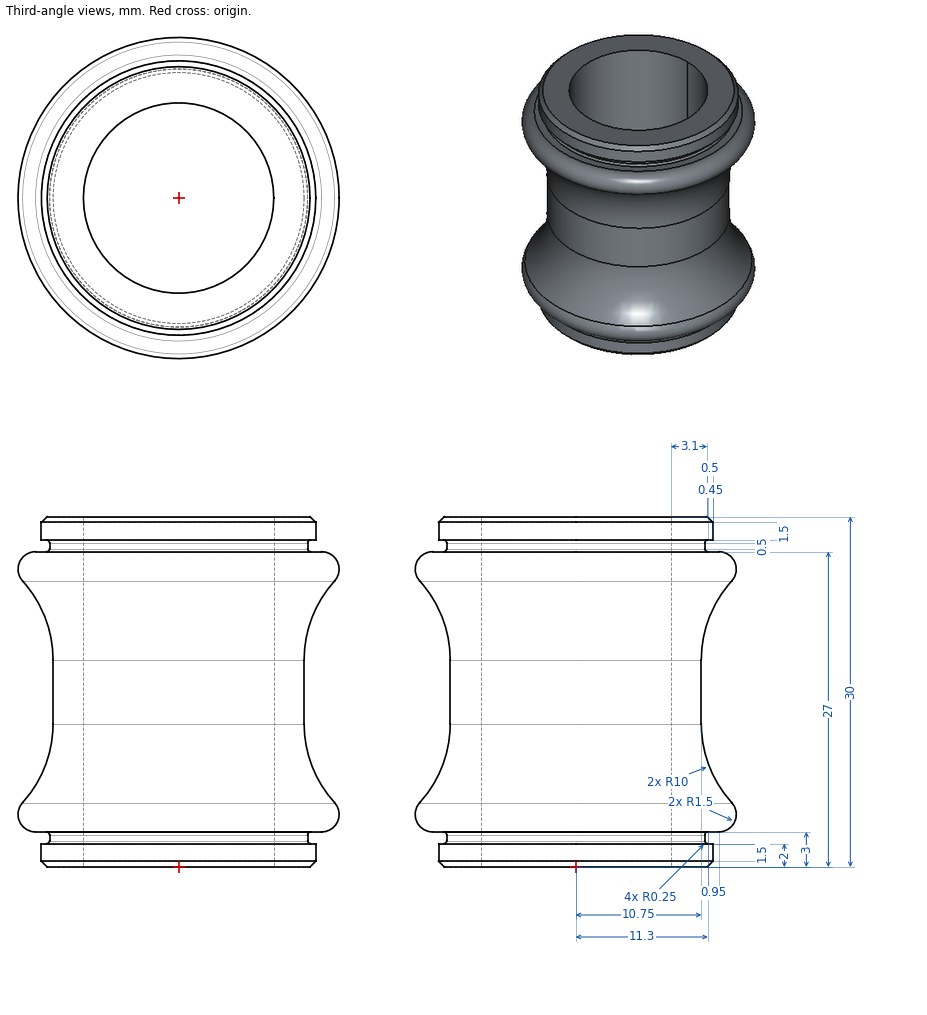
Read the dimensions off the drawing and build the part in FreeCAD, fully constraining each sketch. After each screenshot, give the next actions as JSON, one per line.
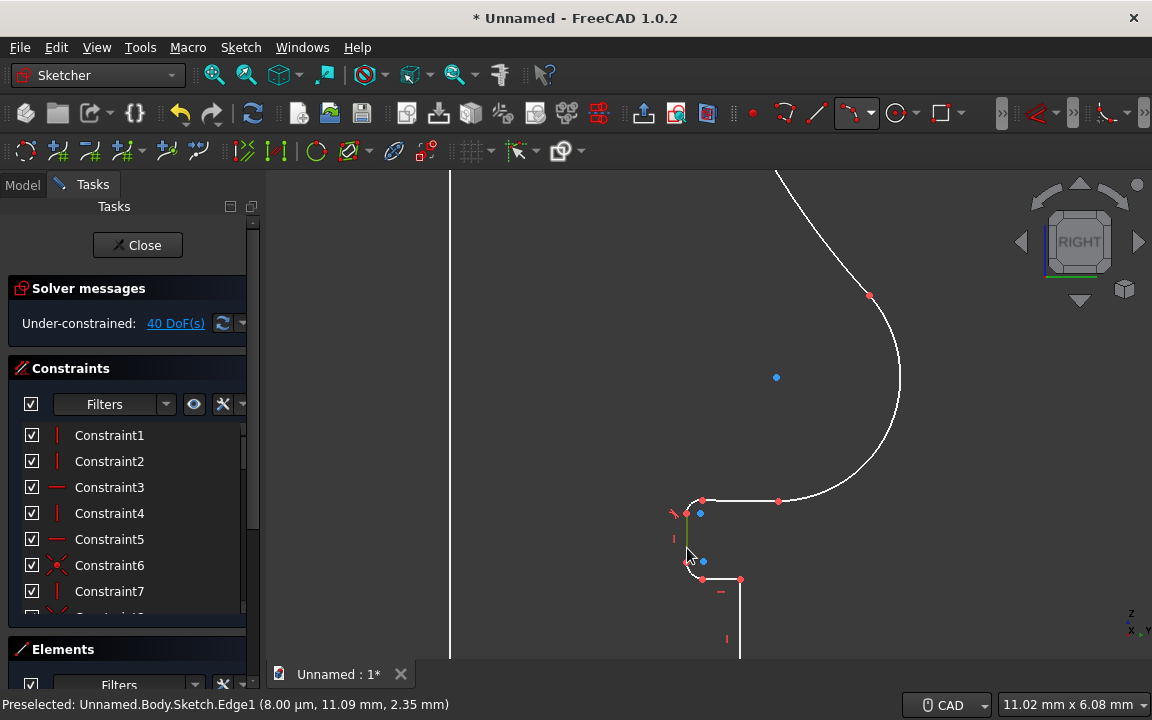
{"action": "left_click", "coordinate": [692, 574]}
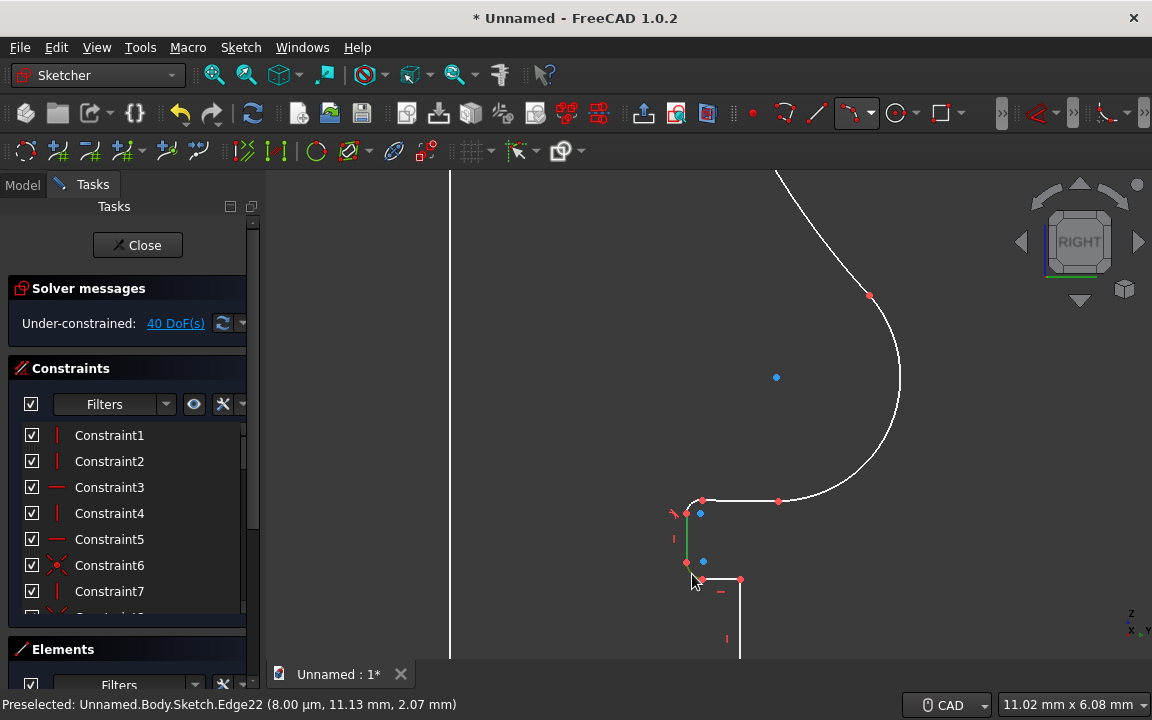
{"action": "key", "text": "t"}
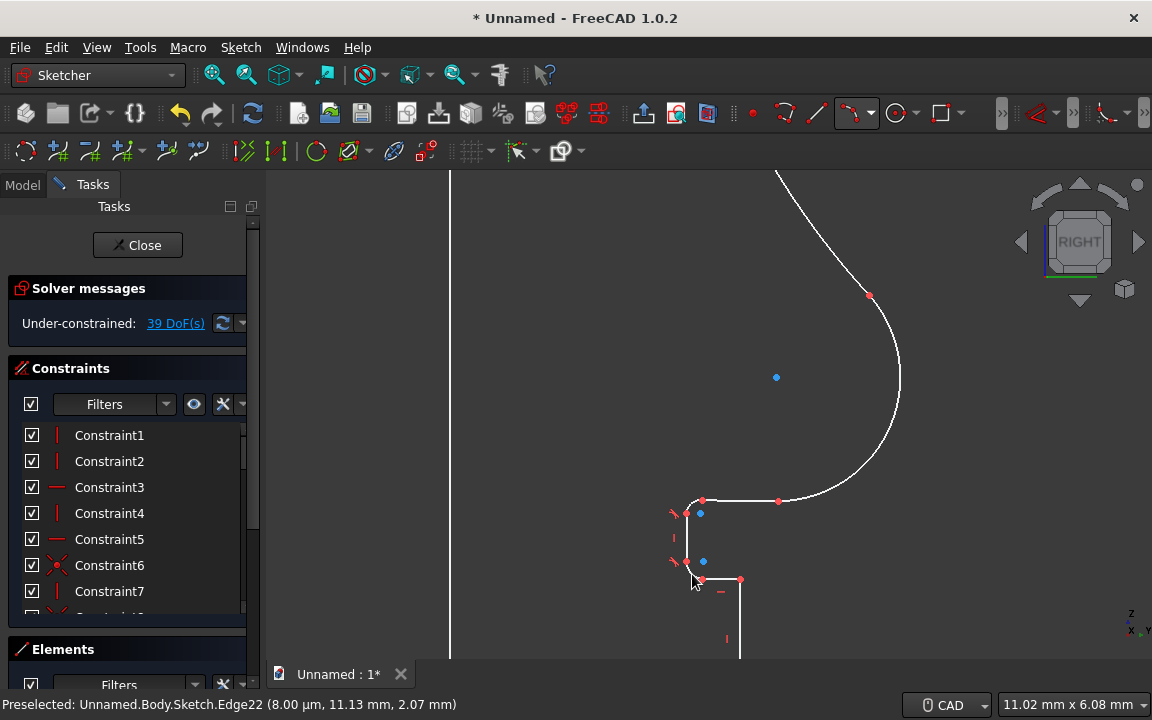
{"action": "left_click", "coordinate": [725, 501]}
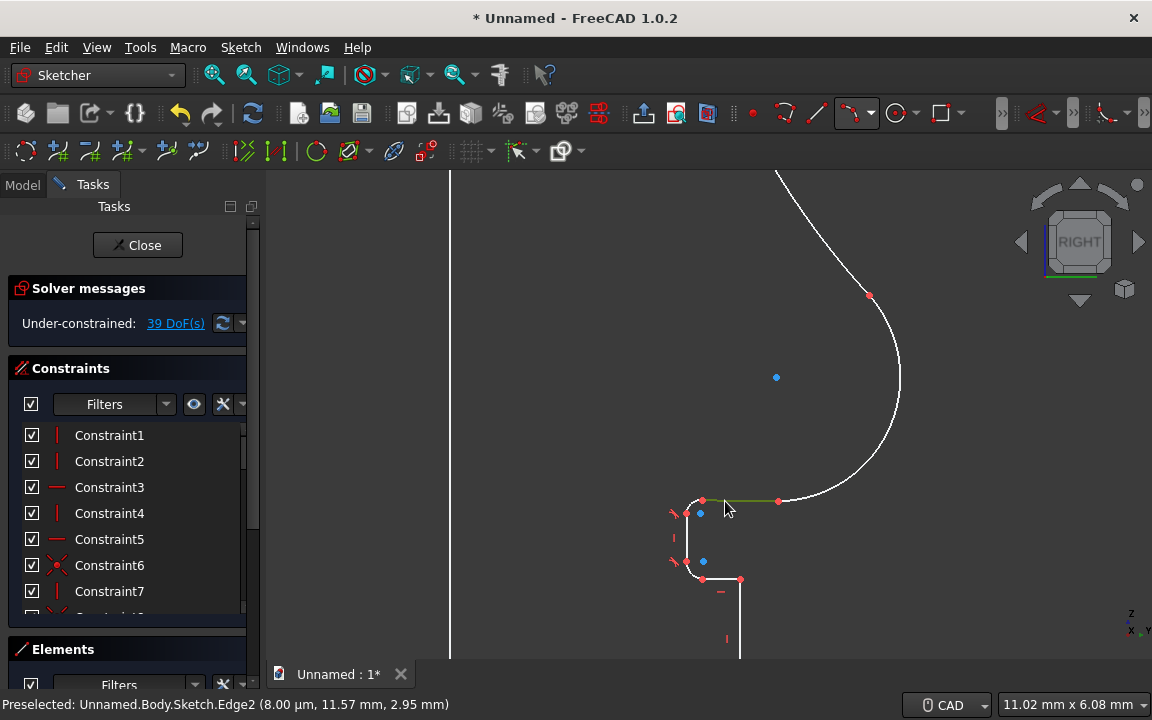
{"action": "left_click", "coordinate": [692, 503]}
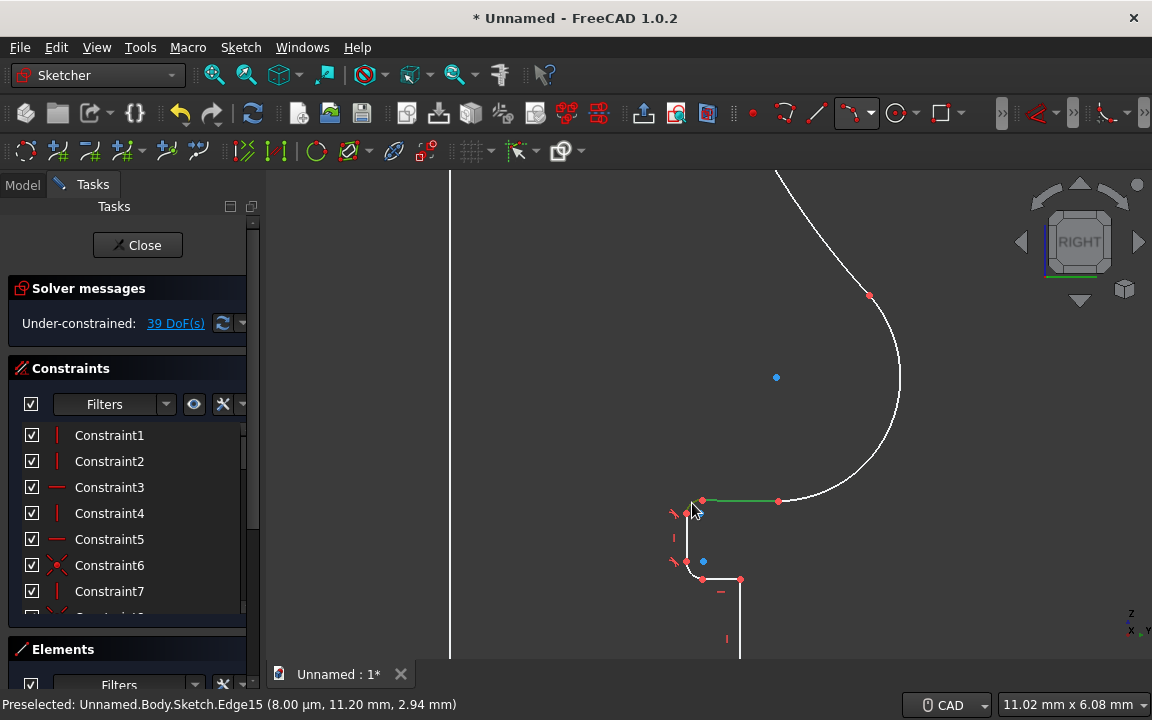
{"action": "key", "text": "t"}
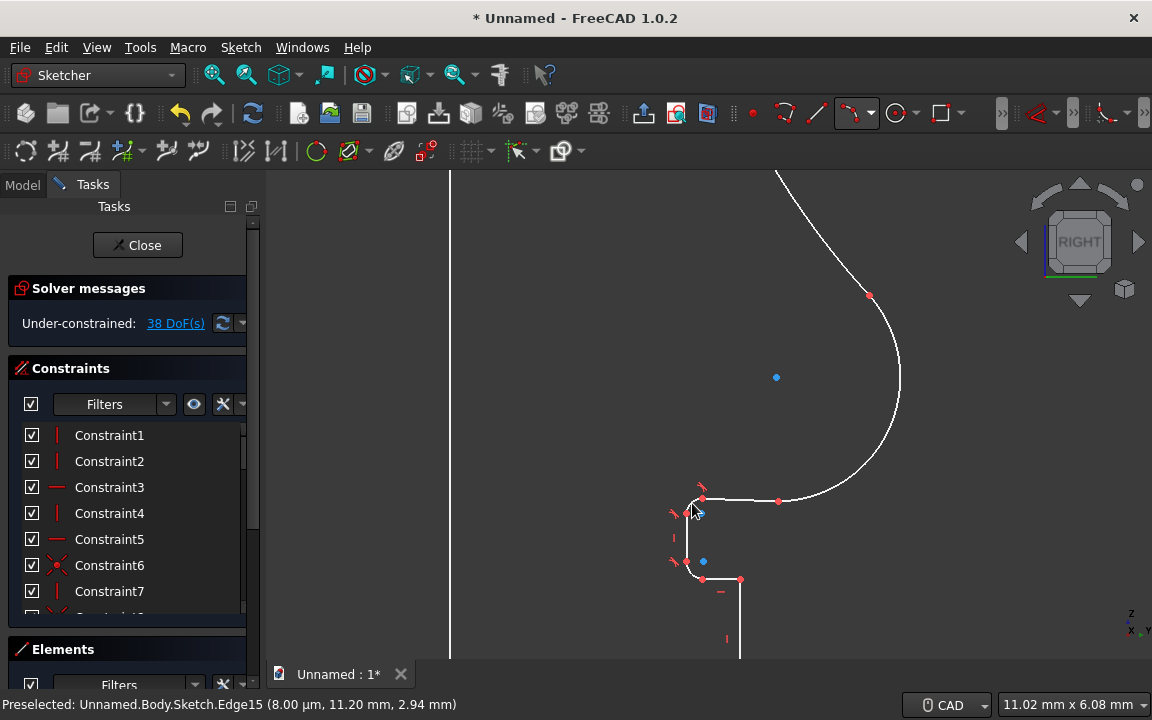
{"action": "left_click", "coordinate": [725, 499]}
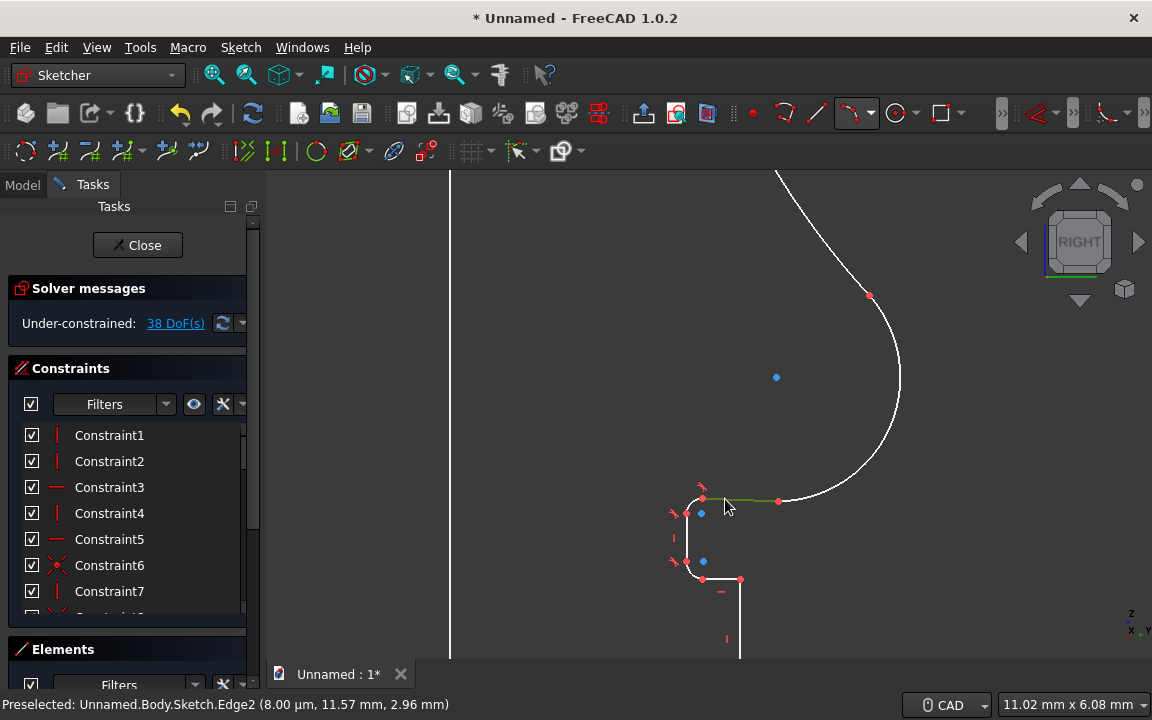
{"action": "scroll", "coordinate": [687, 553], "scroll_direction": "down", "scroll_amount": 10}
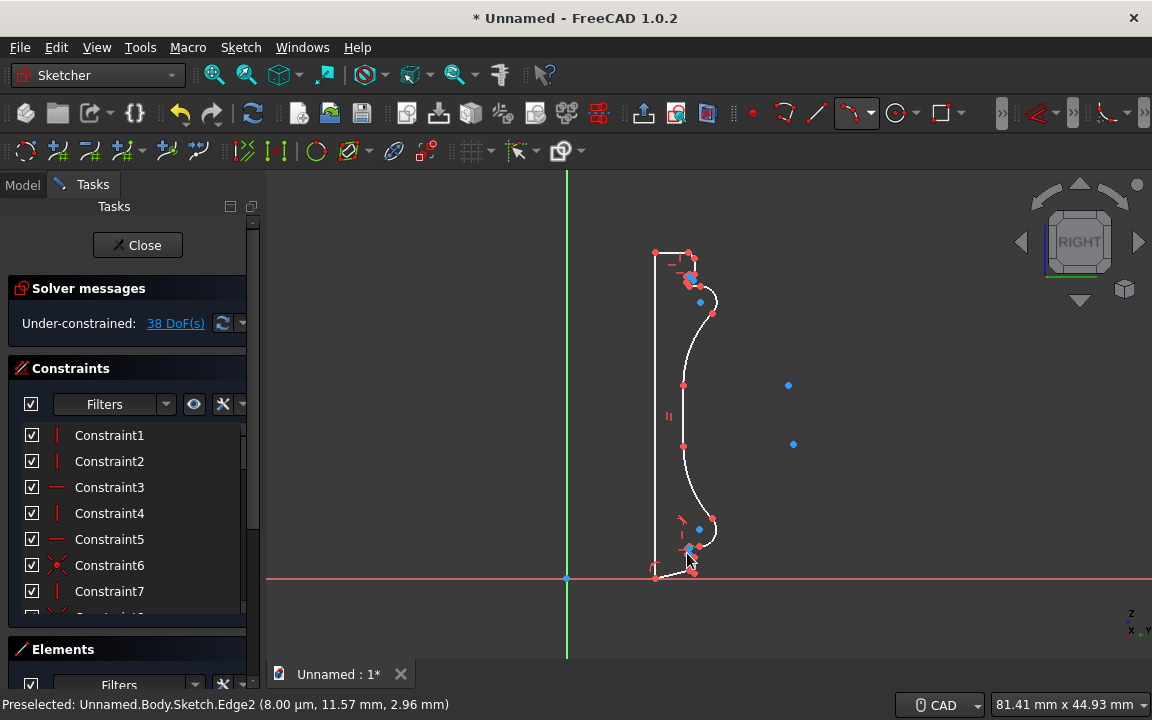
{"action": "scroll", "coordinate": [710, 543], "scroll_direction": "up", "scroll_amount": 2}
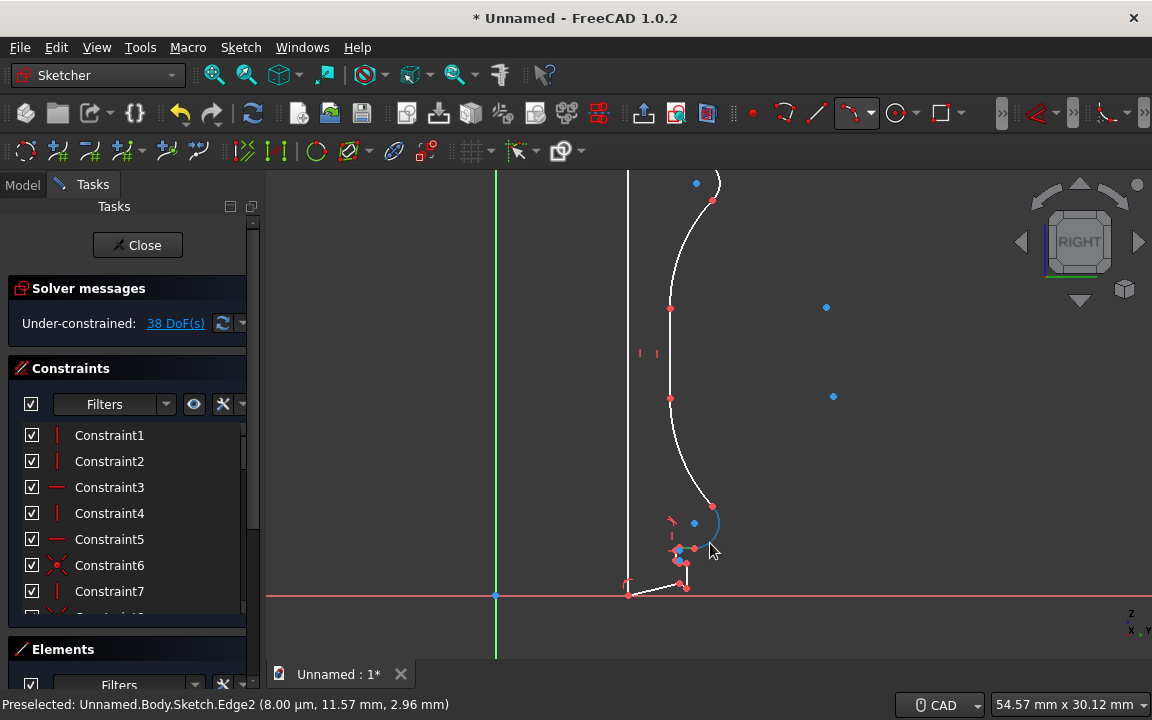
{"action": "left_click", "coordinate": [710, 542]}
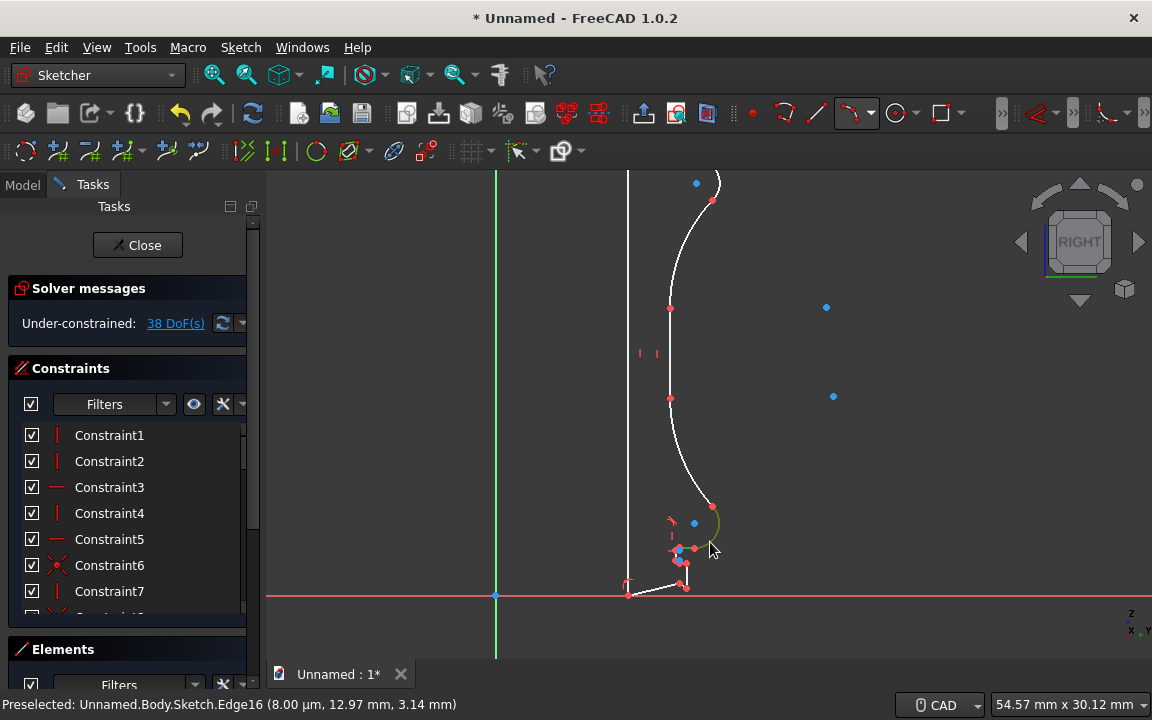
{"action": "key", "text": "t"}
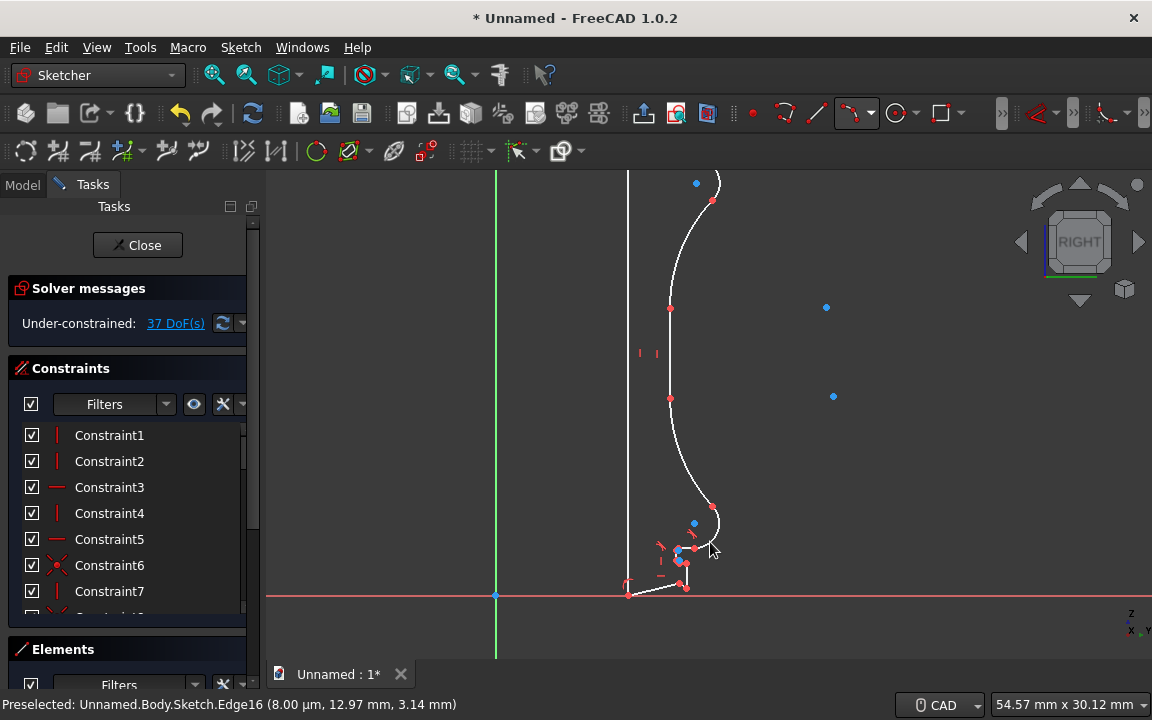
{"action": "left_click", "coordinate": [670, 371]}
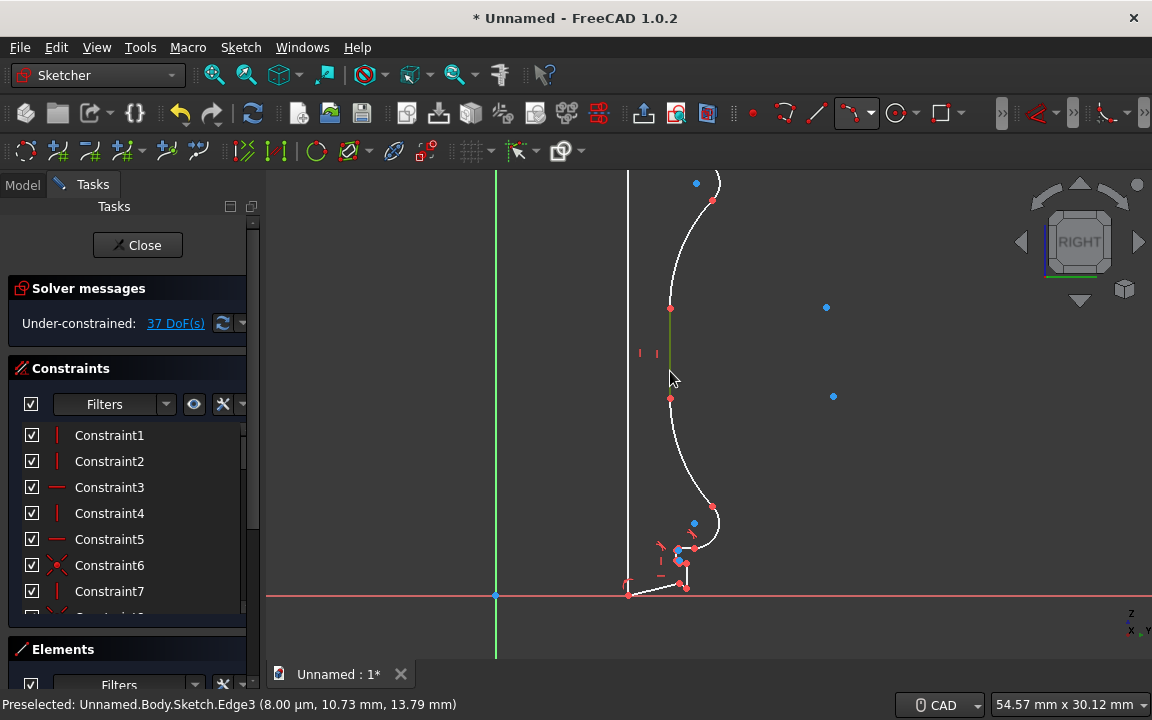
{"action": "left_click", "coordinate": [674, 434]}